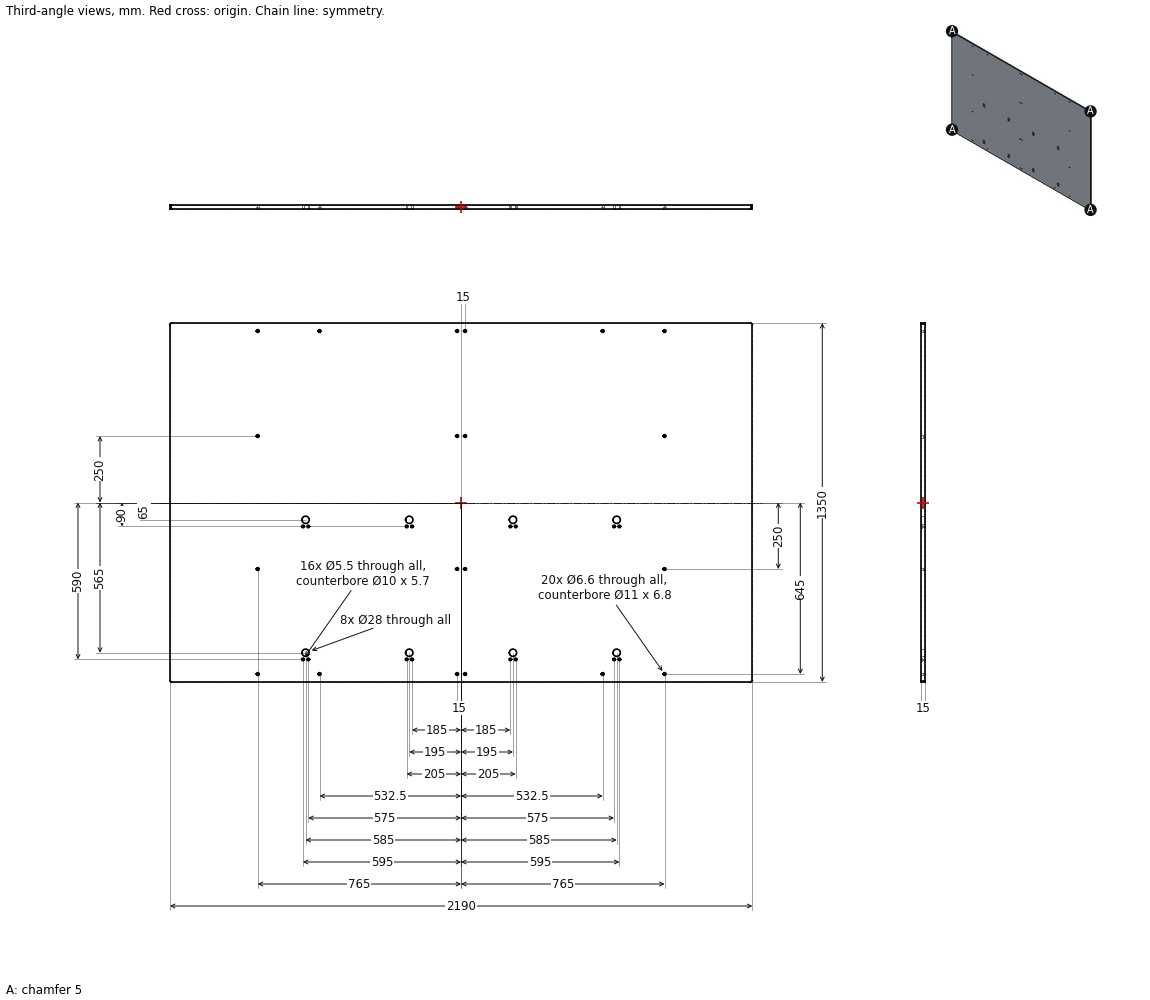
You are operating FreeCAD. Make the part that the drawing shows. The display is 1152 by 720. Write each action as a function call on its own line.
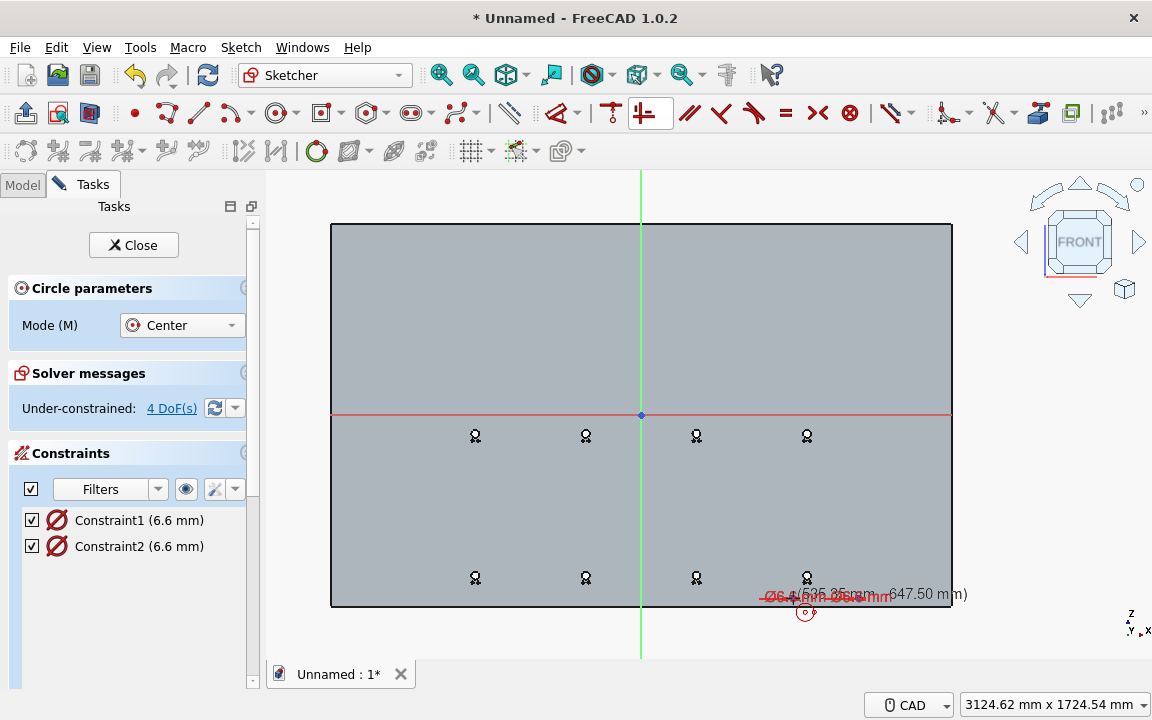
scroll(858, 486, up, 16)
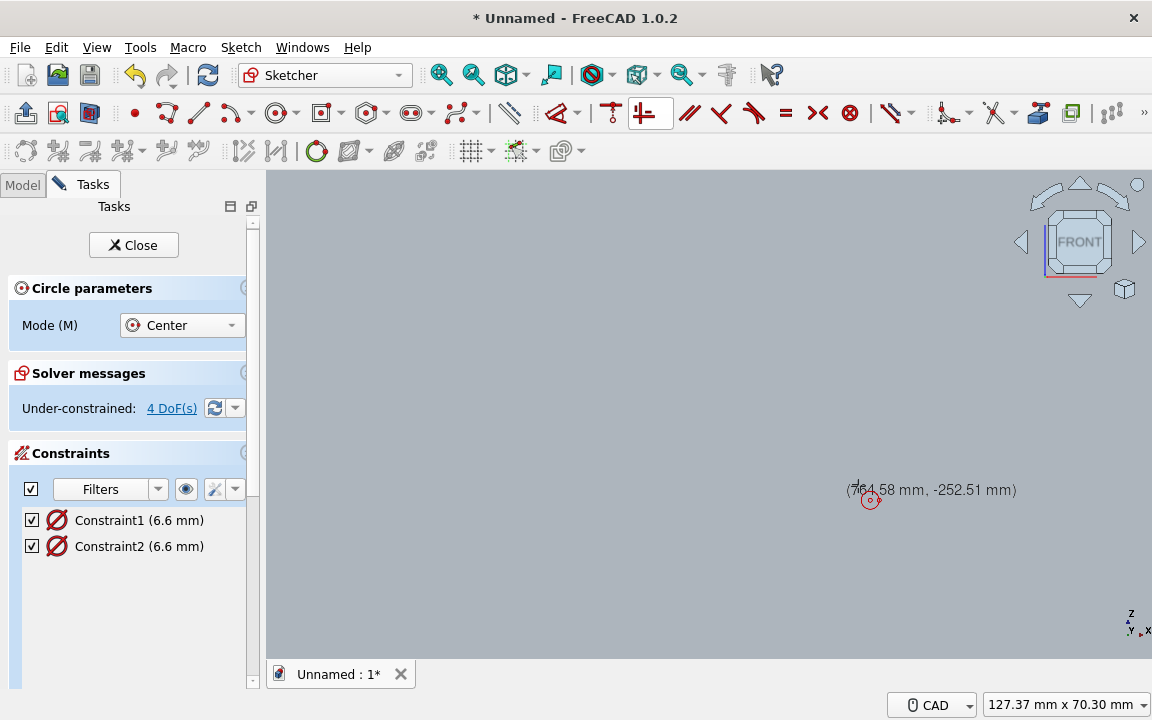
scroll(858, 486, down, 16)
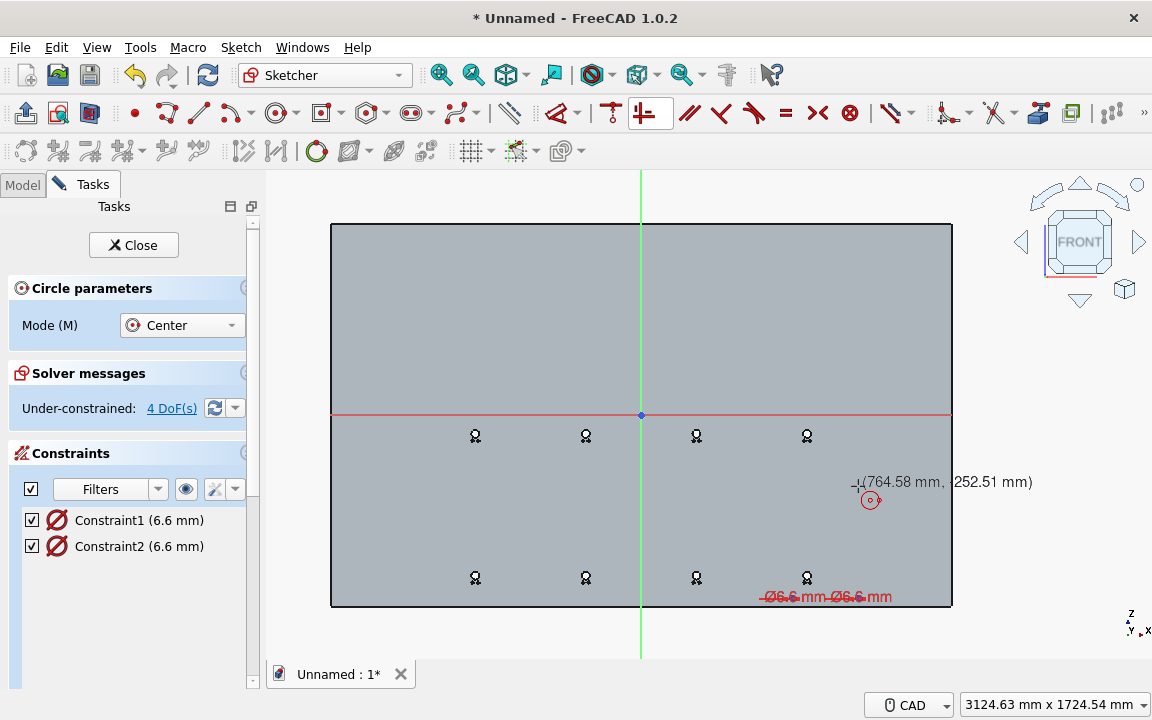
click(858, 486)
move(859, 486)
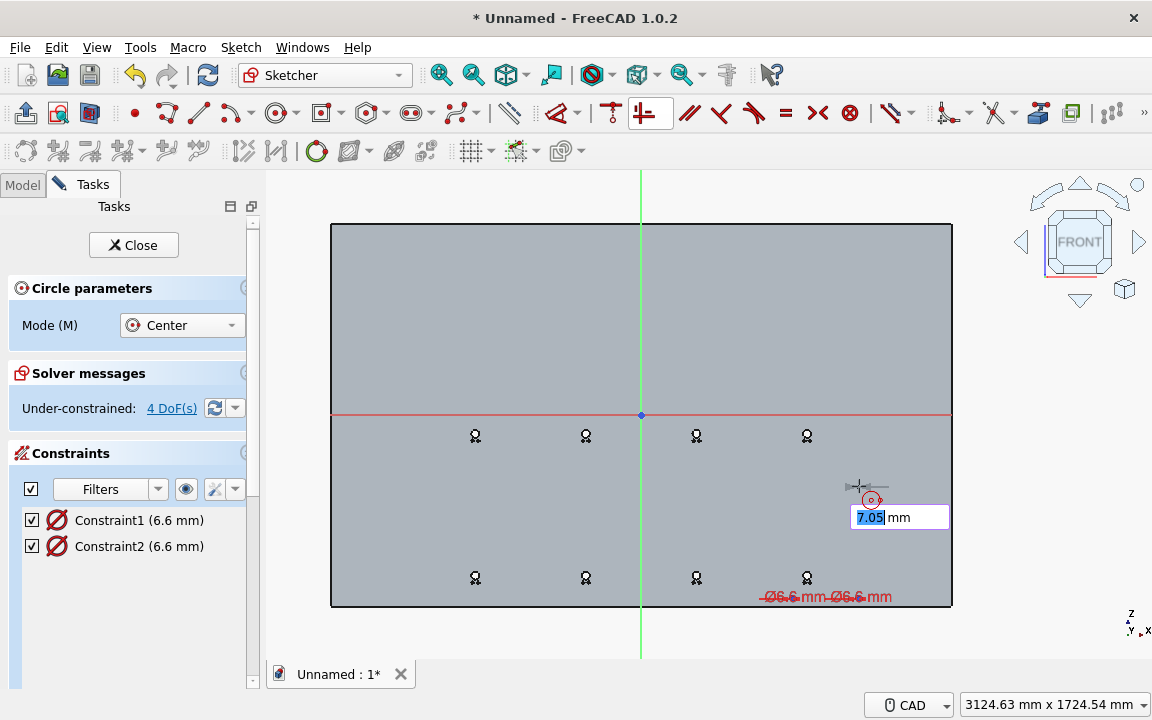
text(6.6)
key(Return)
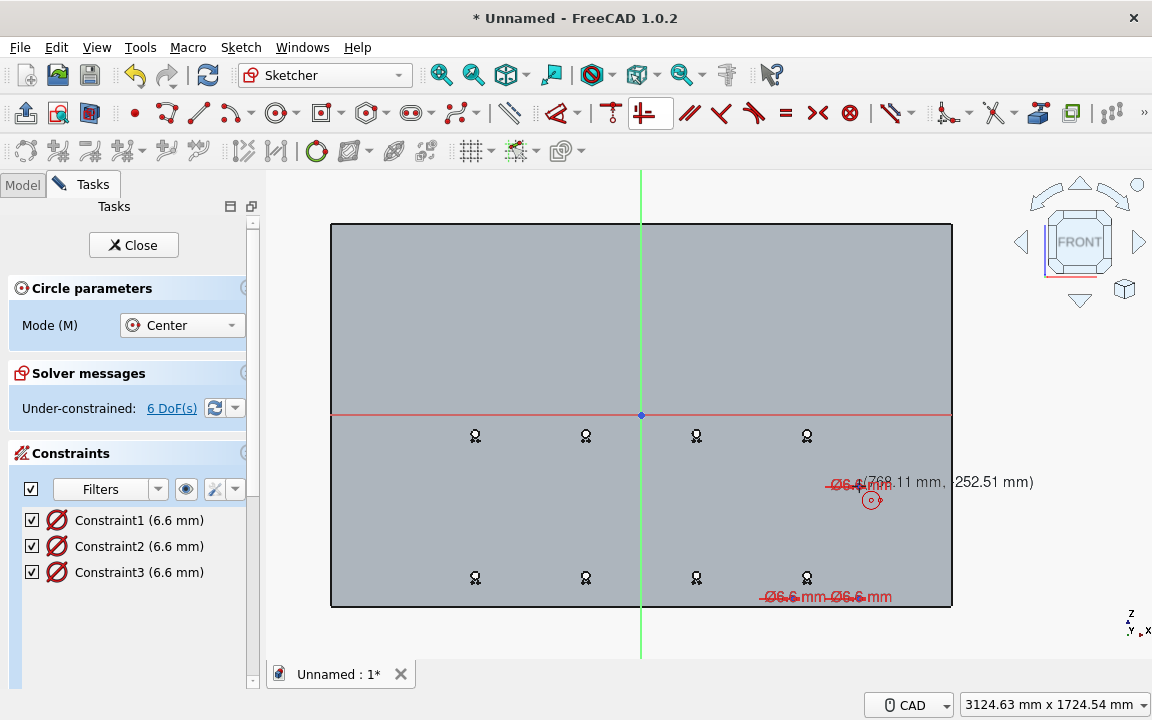
scroll(637, 598, up, 16)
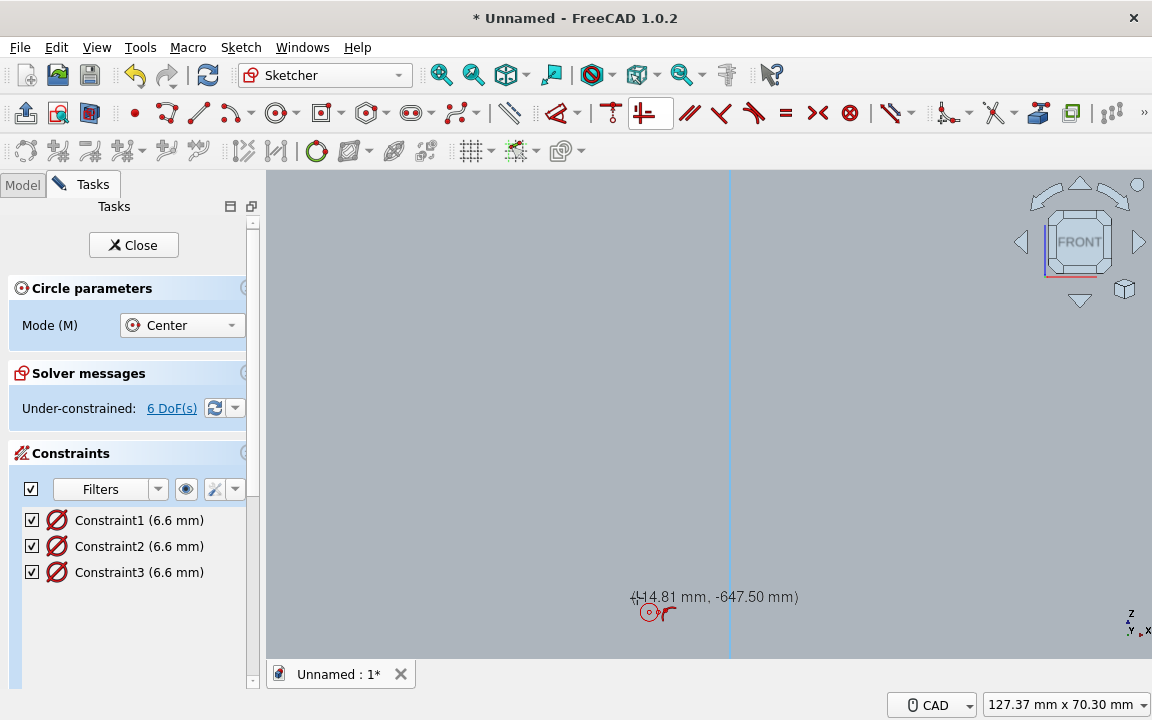
scroll(637, 598, down, 16)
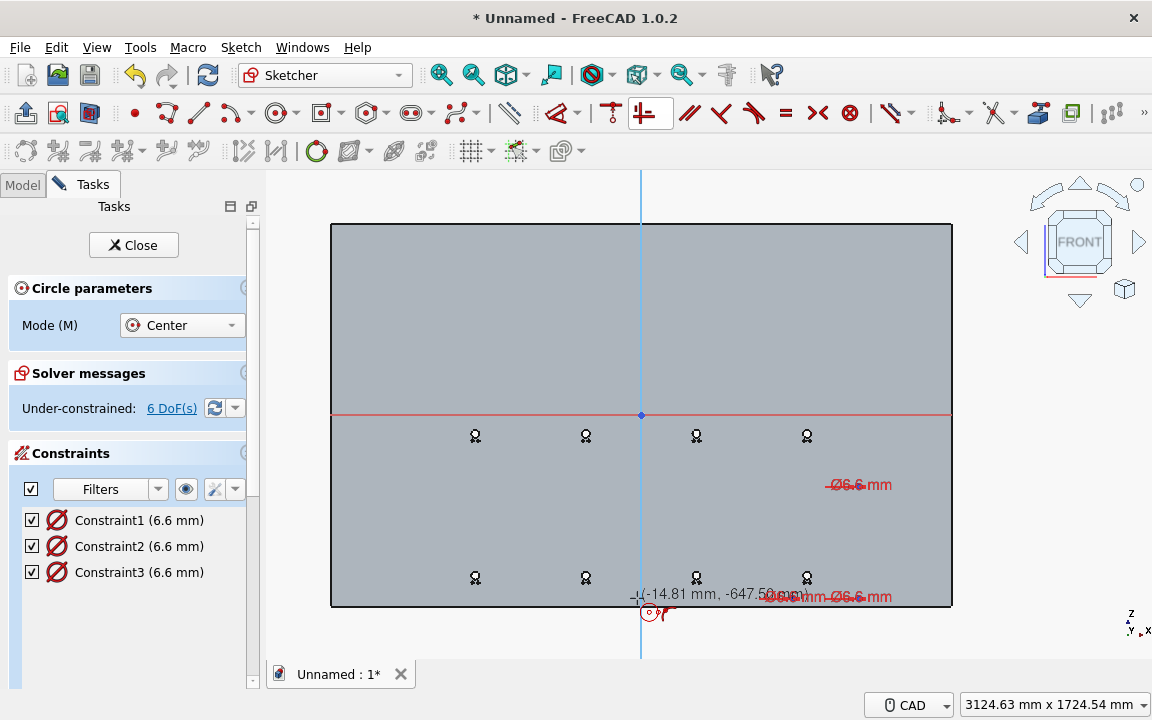
scroll(637, 598, up, 7)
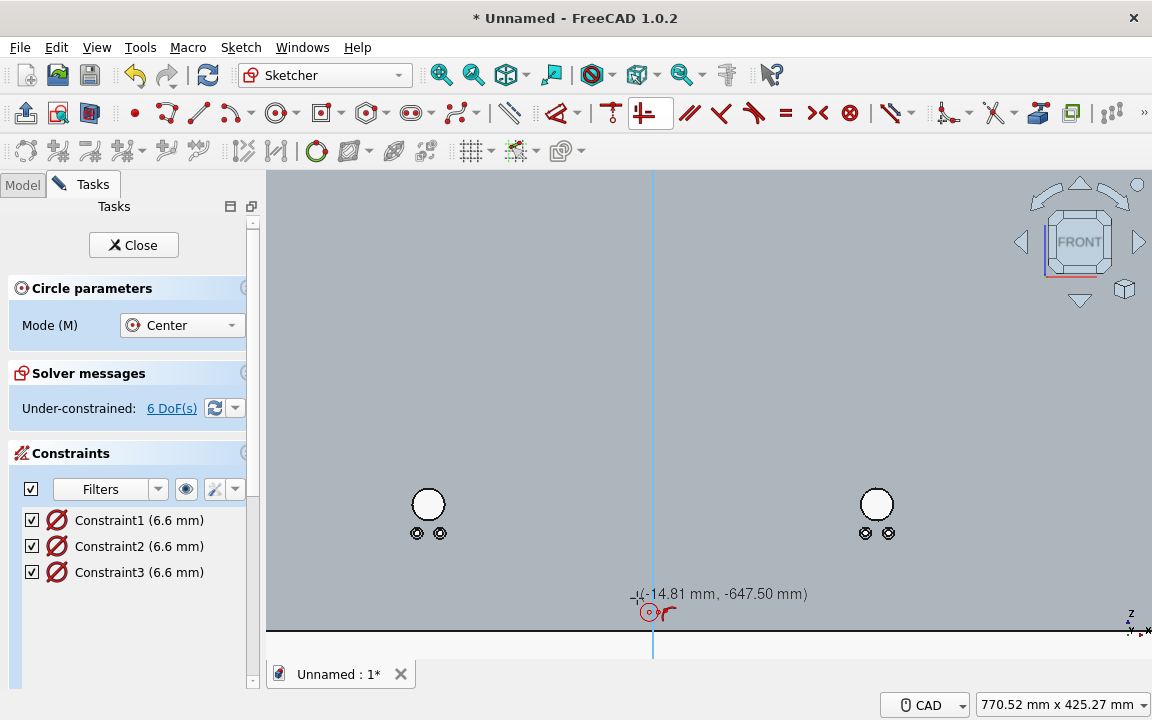
click(636, 597)
move(638, 594)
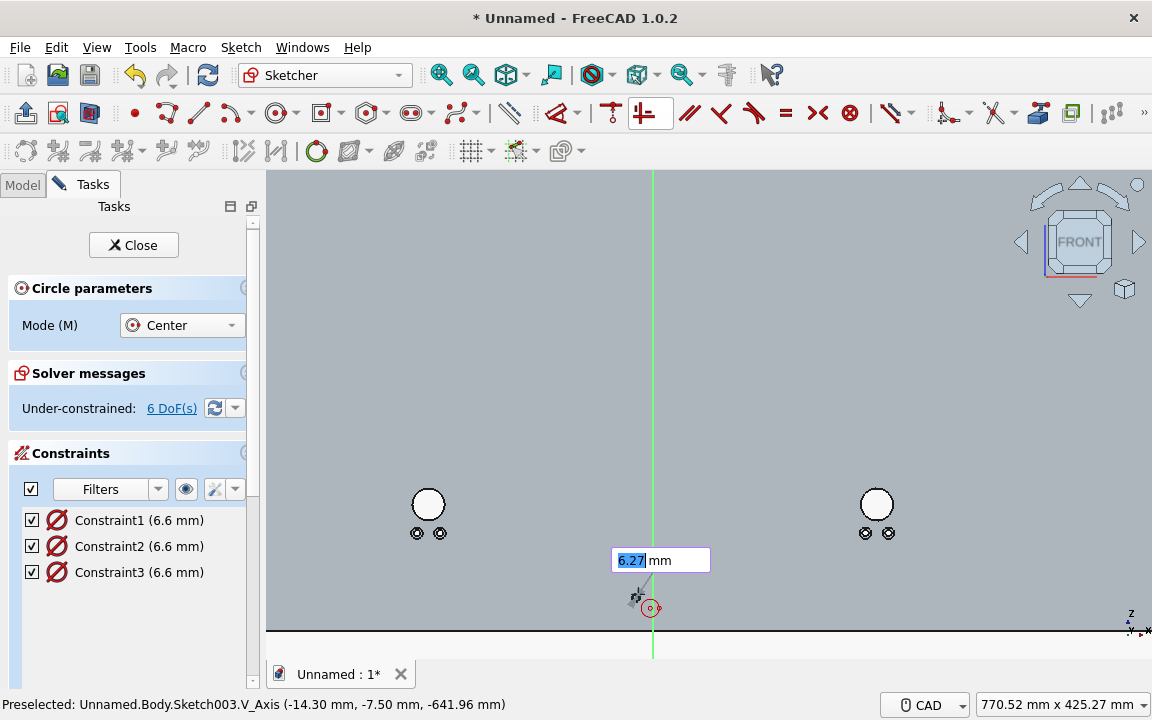
text(6.6)
key(Return)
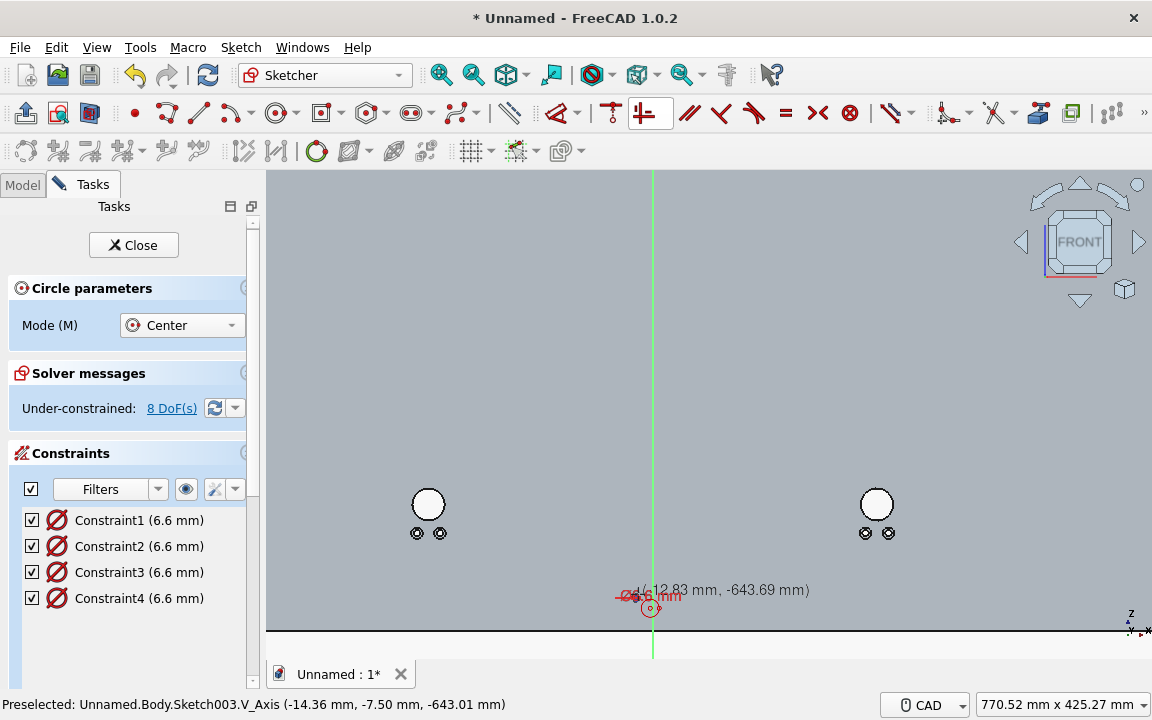
scroll(637, 556, down, 8)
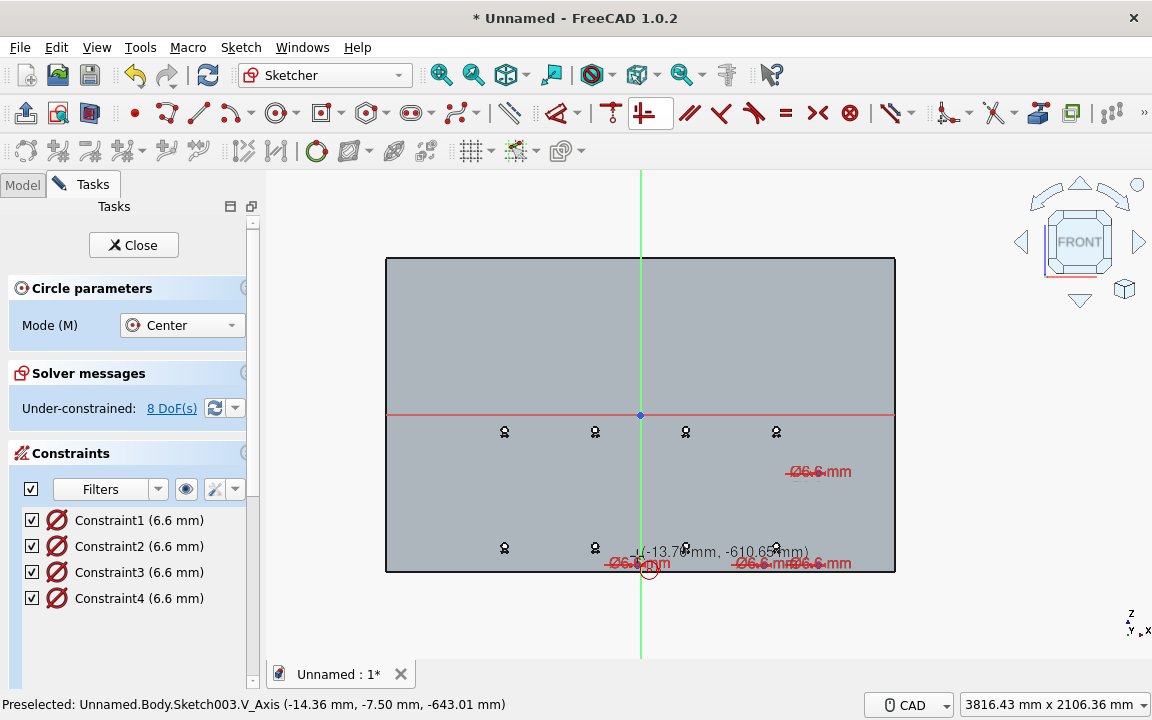
scroll(637, 473, up, 17)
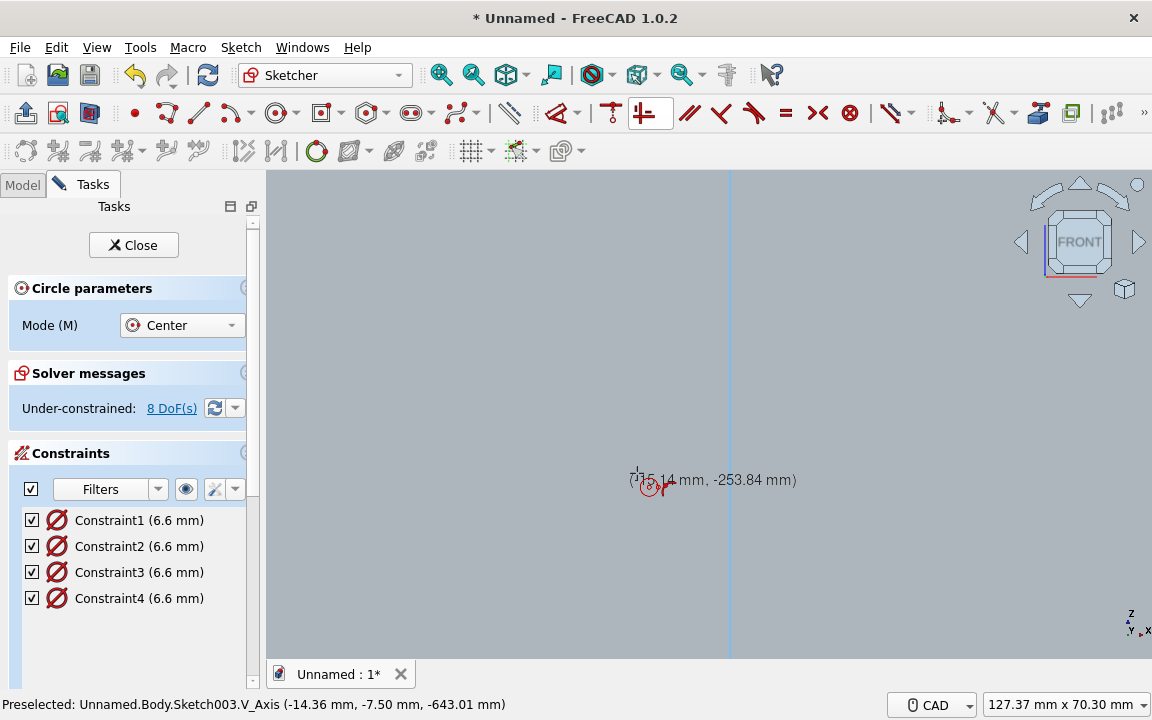
scroll(637, 487, down, 16)